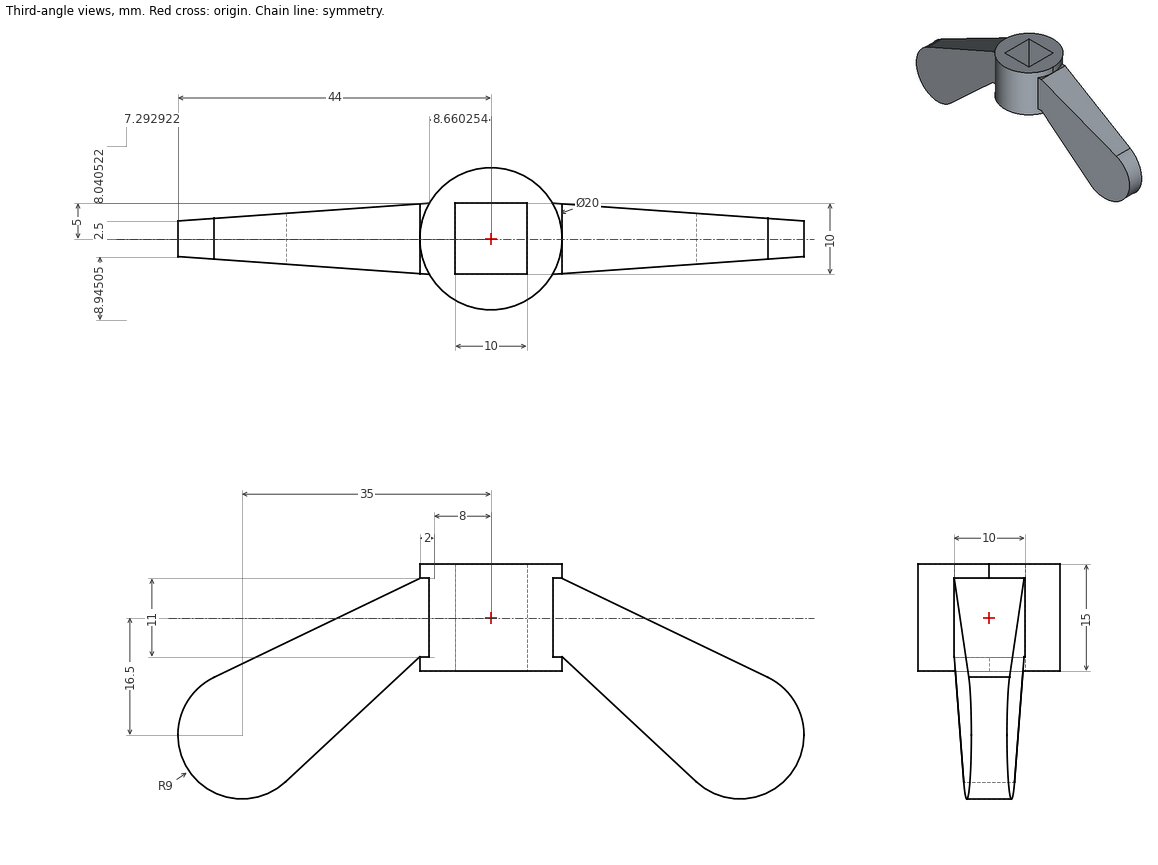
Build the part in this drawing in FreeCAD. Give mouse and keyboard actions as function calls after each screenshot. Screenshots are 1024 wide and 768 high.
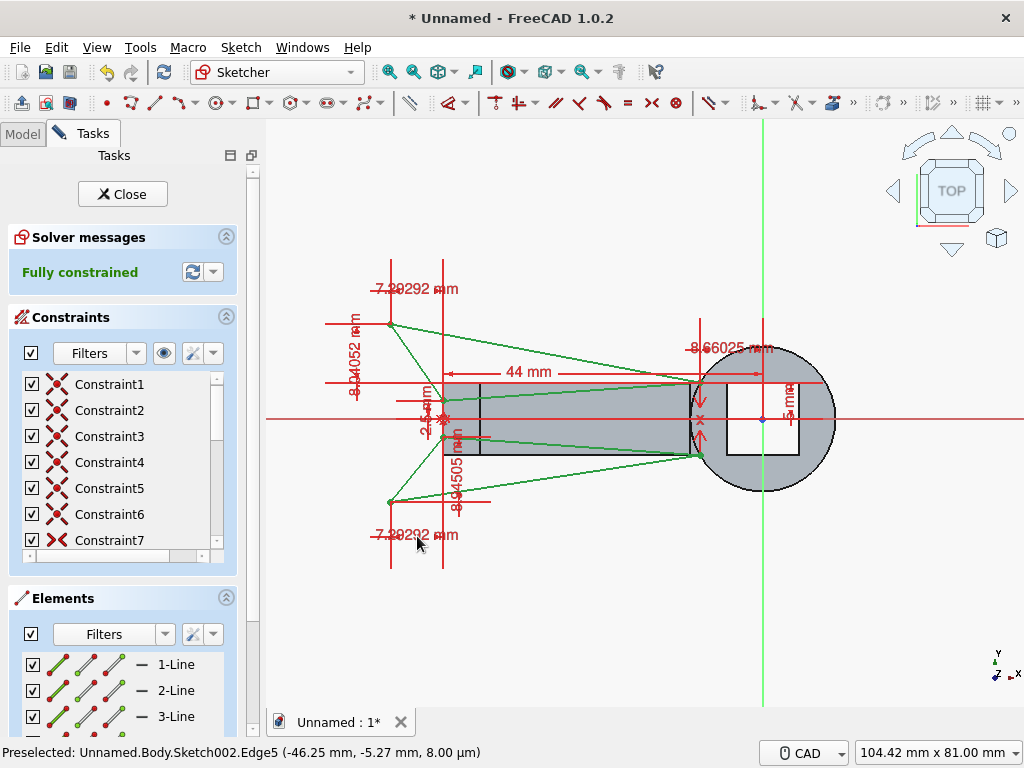
click(123, 194)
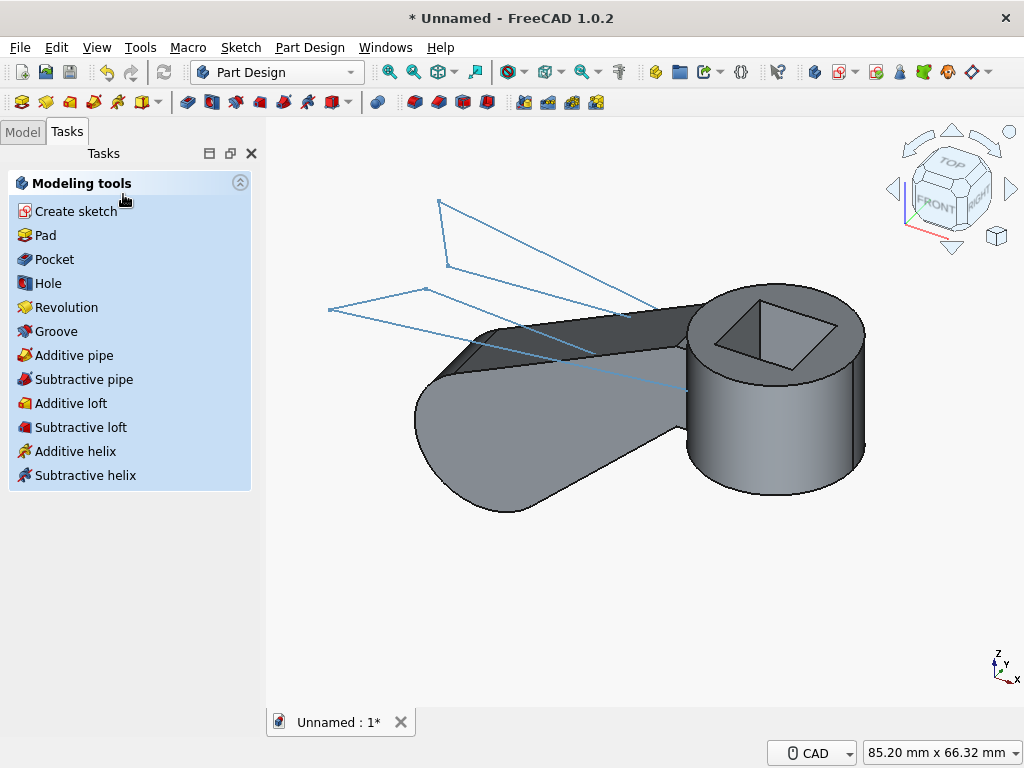
click(188, 102)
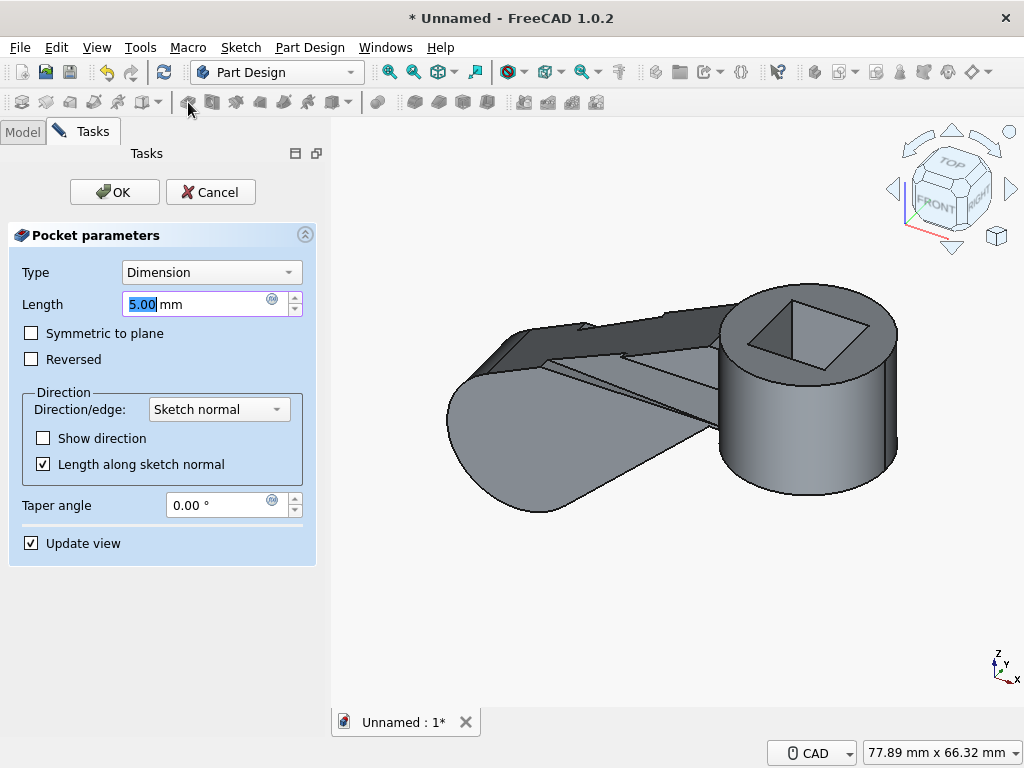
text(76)
key(Tab)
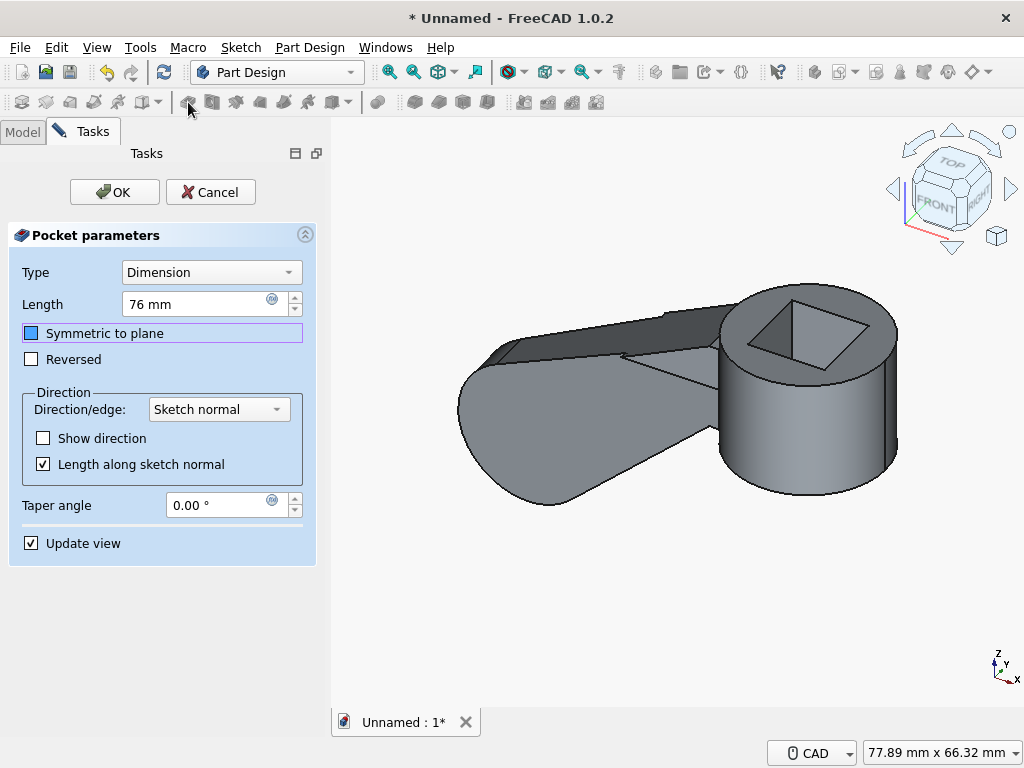
click(30, 333)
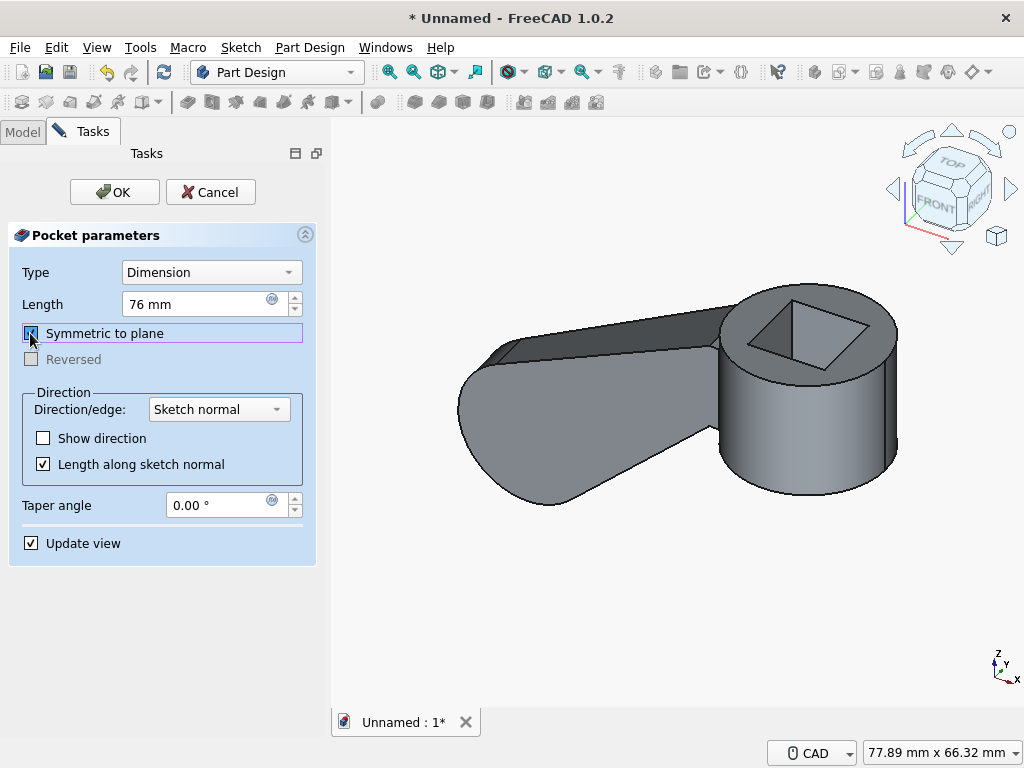
click(115, 192)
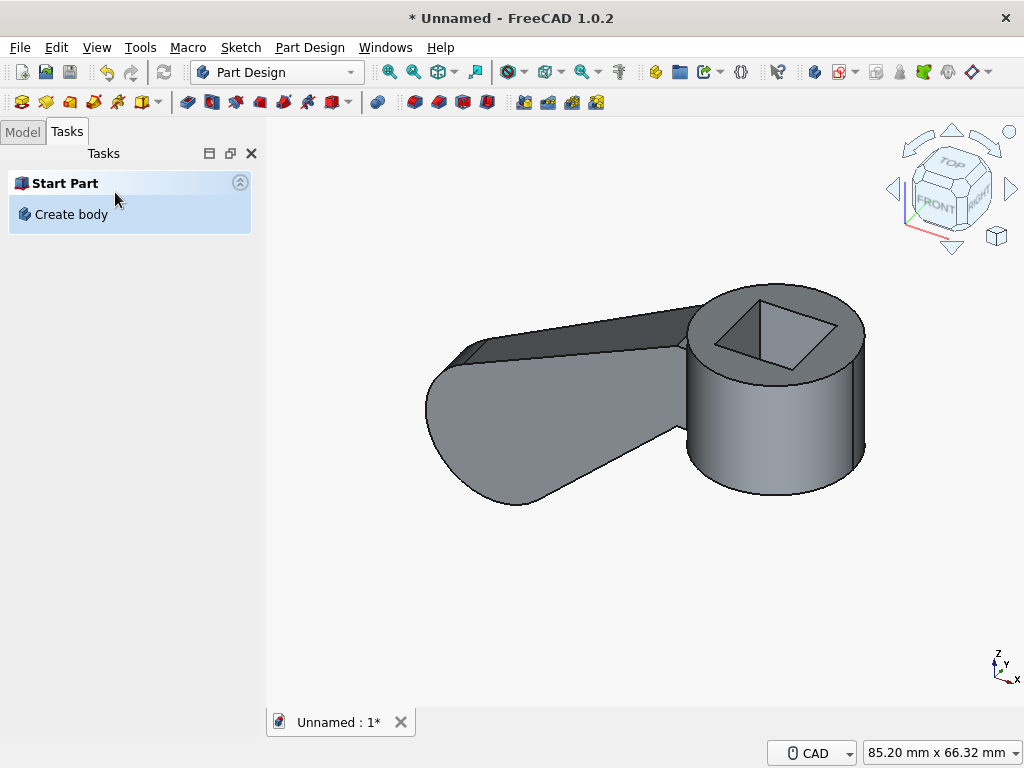
click(23, 131)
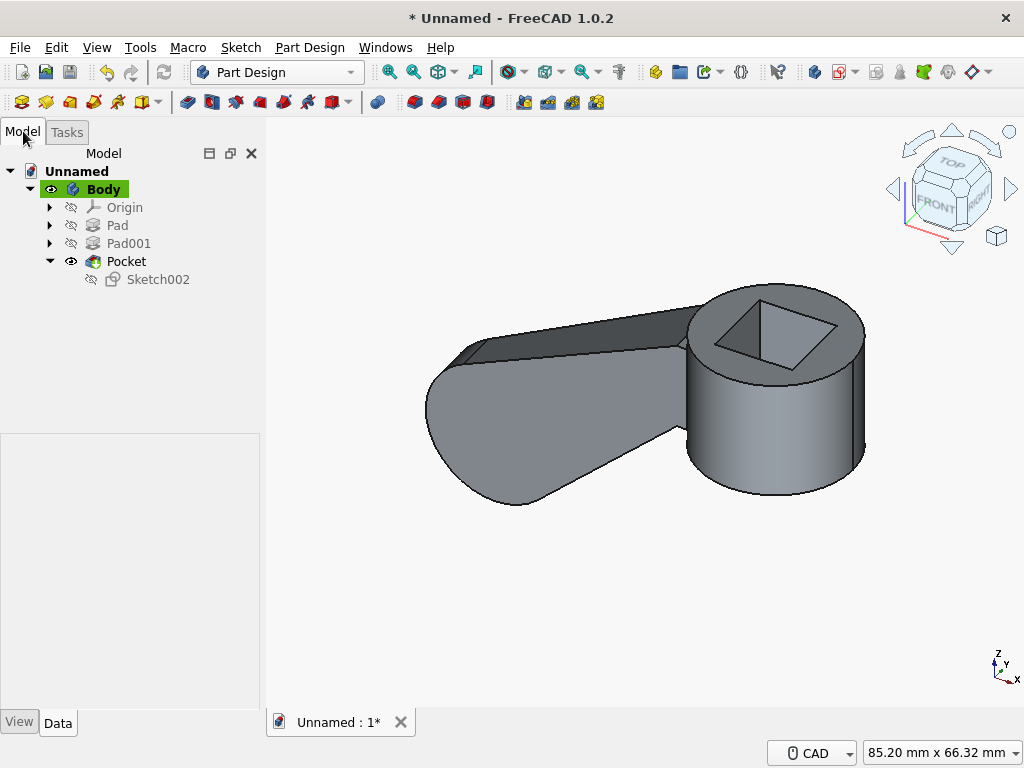
click(116, 243)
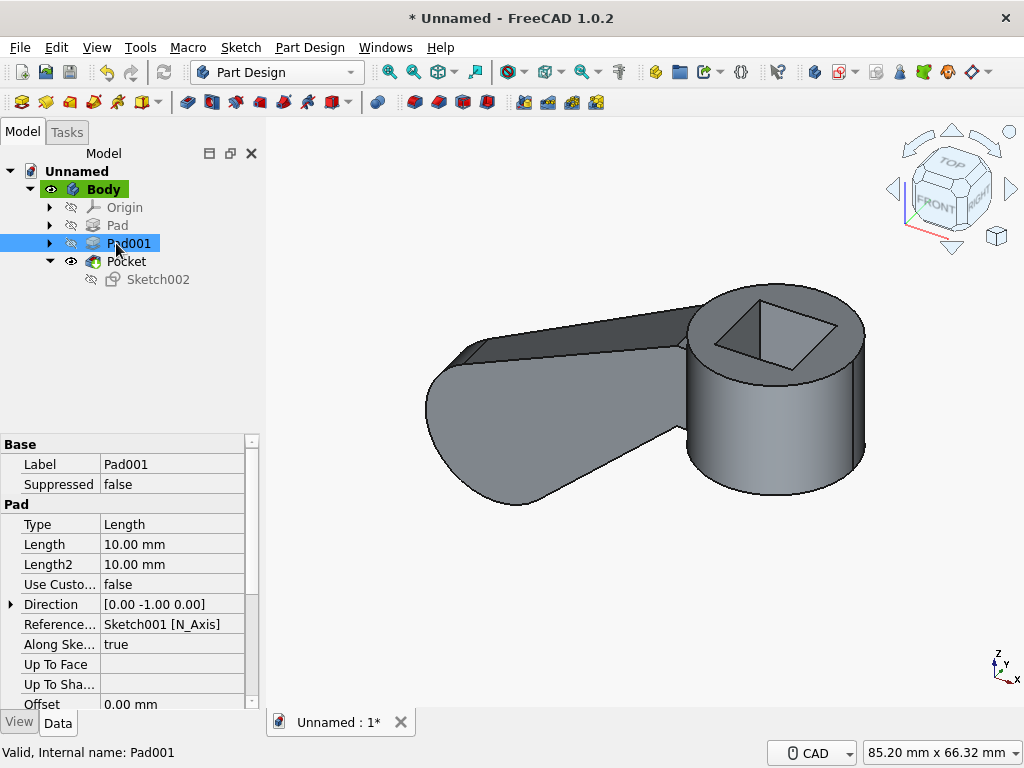
click(116, 261, ctrl)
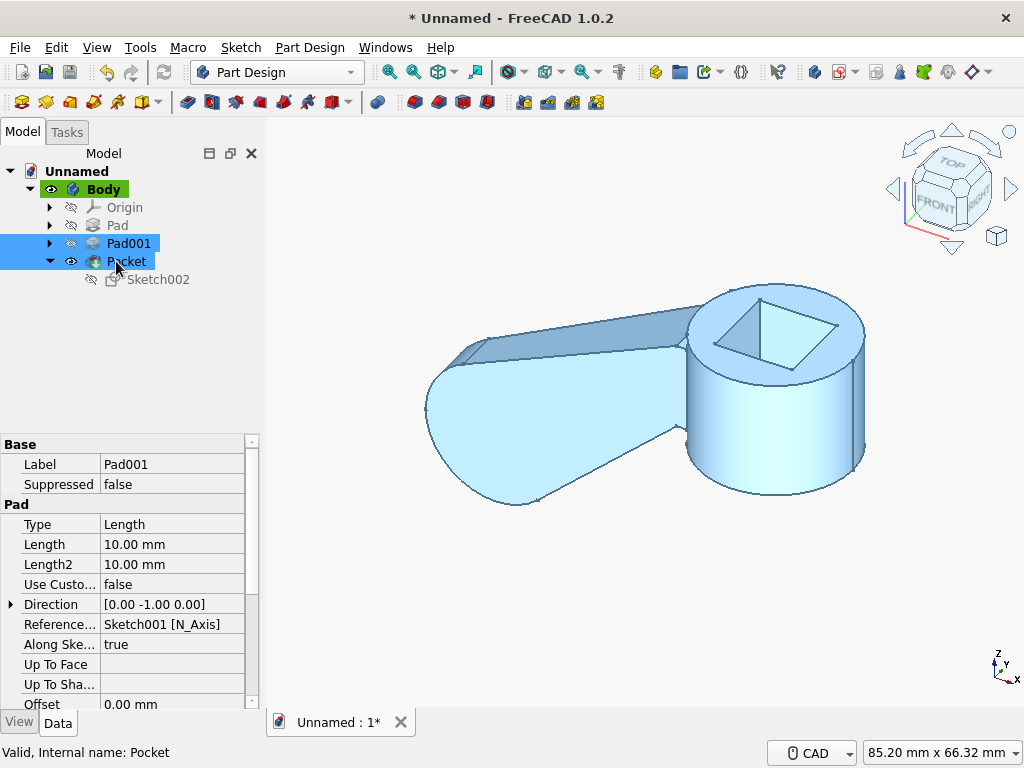
click(524, 102)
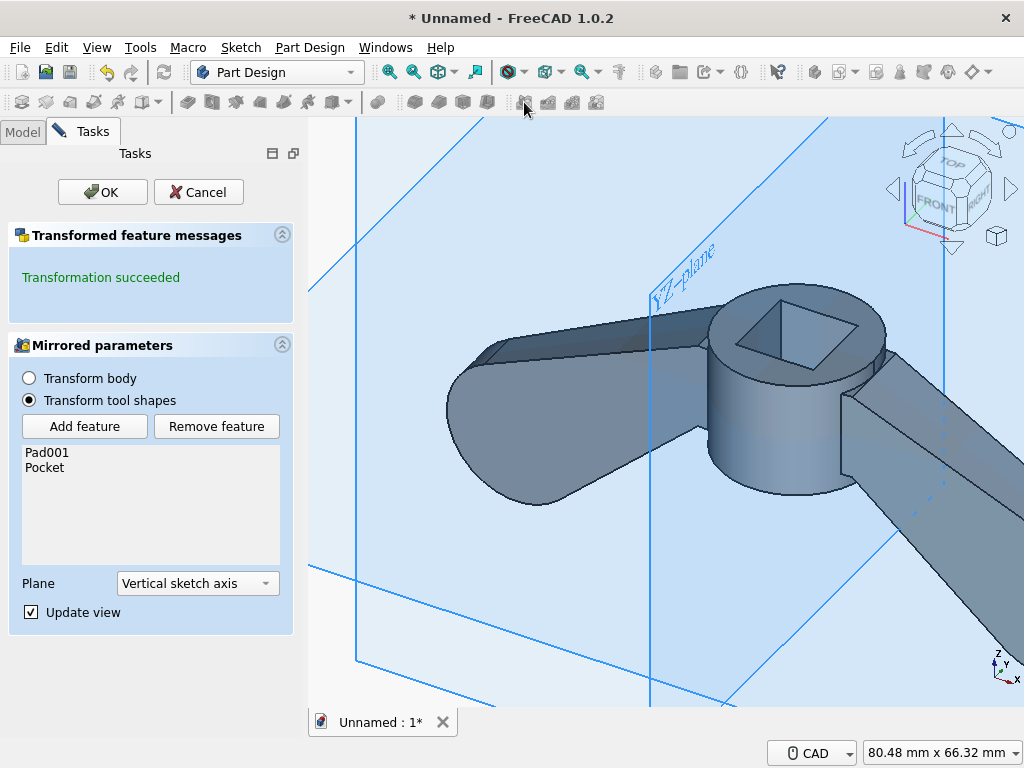
click(198, 584)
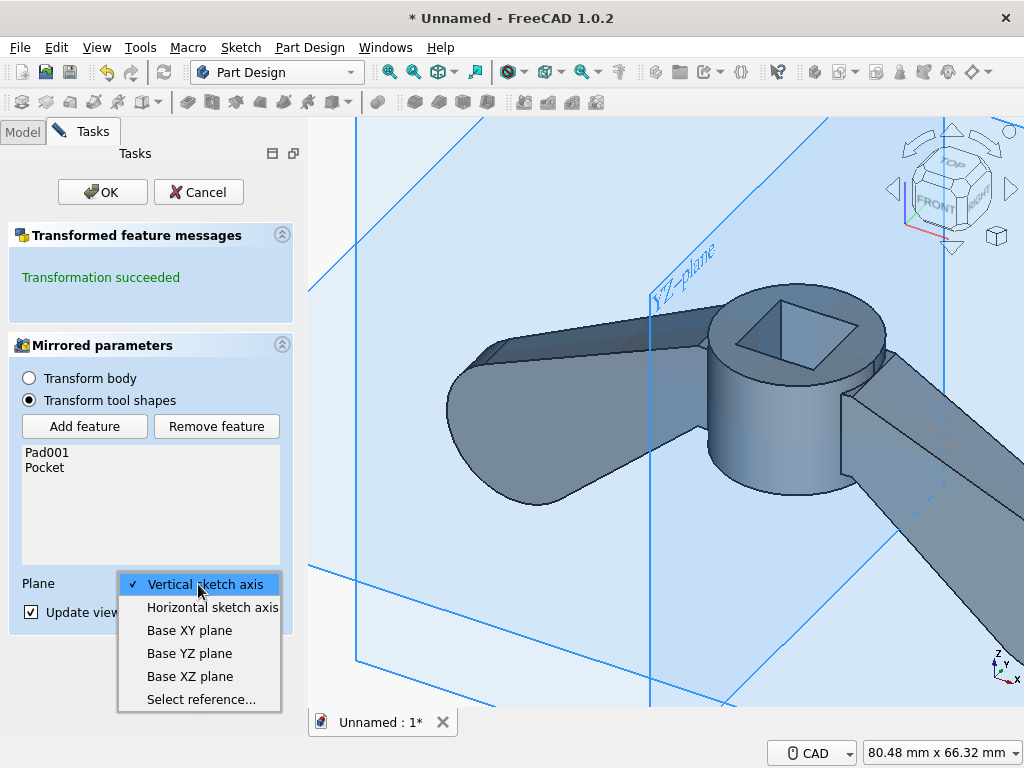
click(198, 654)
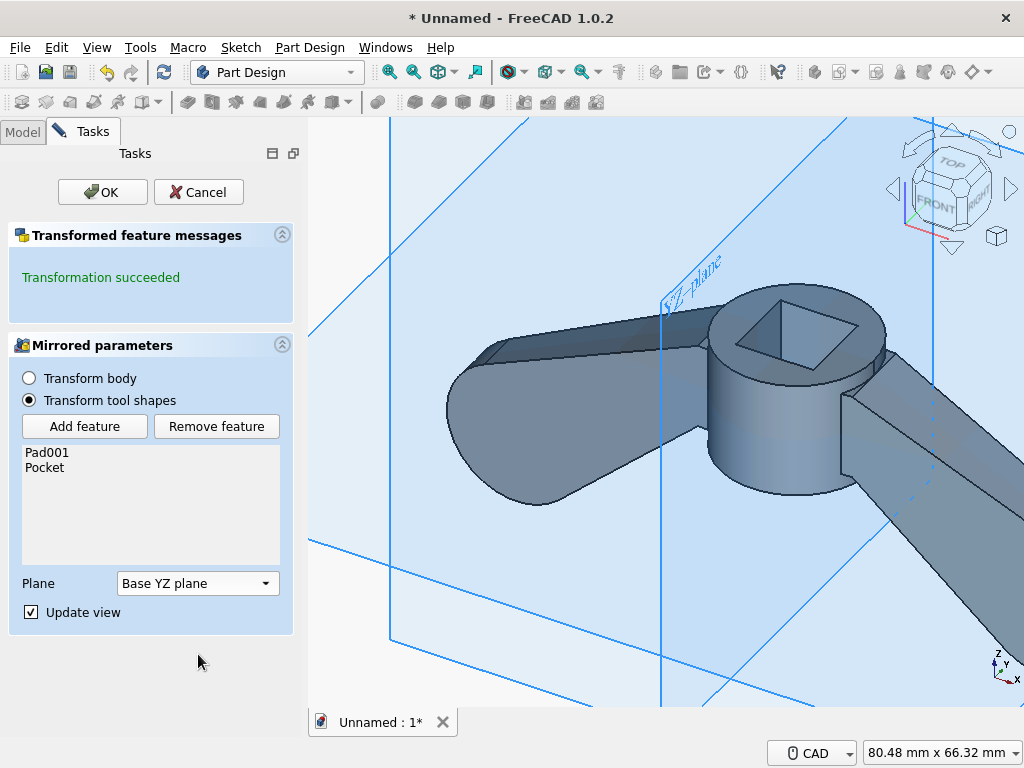
click(103, 192)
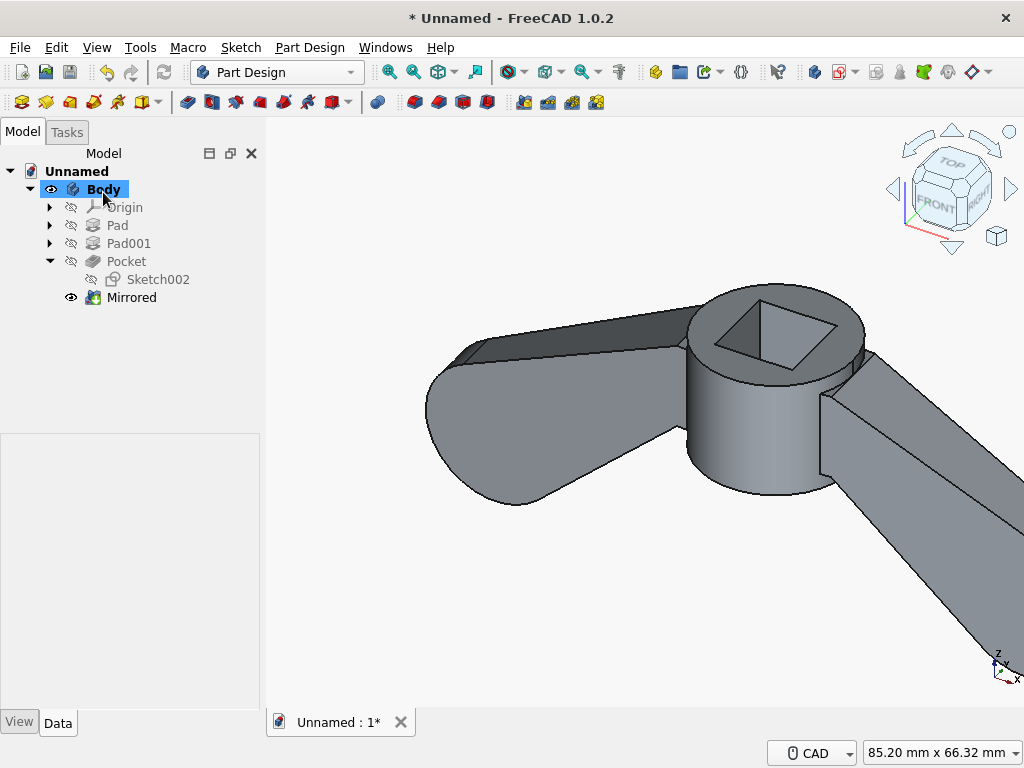
key(0)